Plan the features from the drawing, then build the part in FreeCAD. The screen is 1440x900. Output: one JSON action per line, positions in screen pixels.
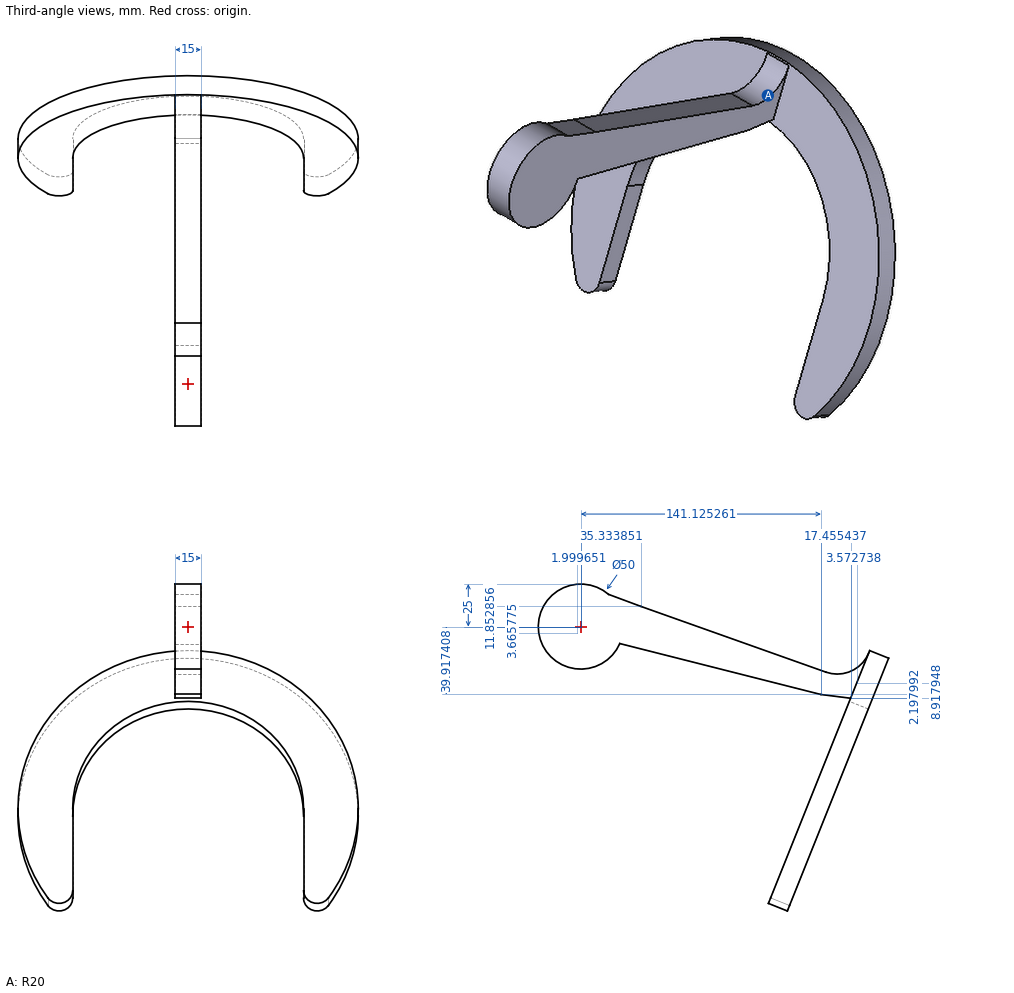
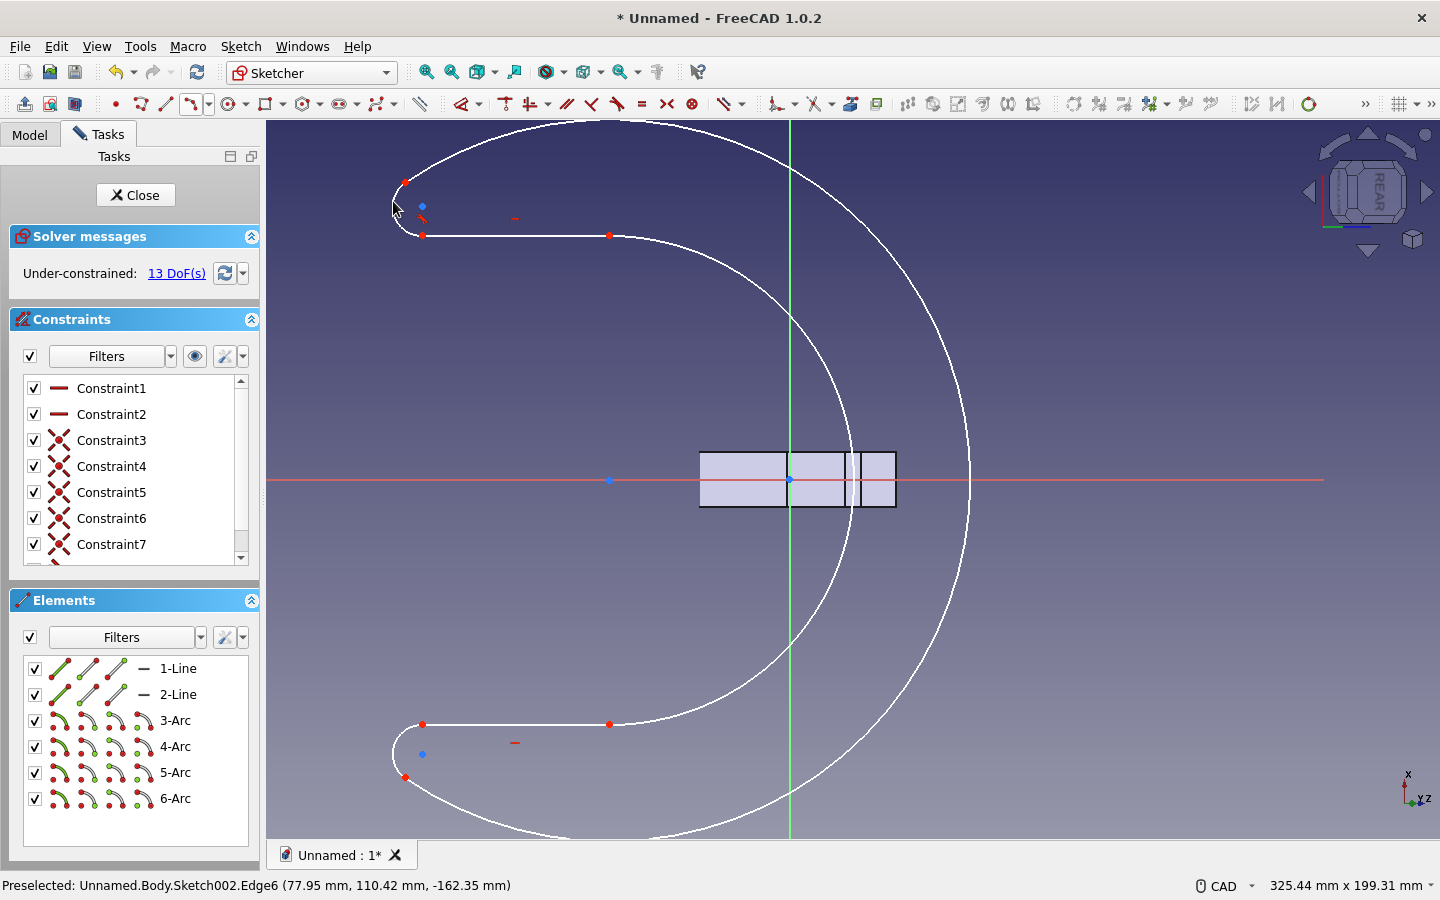
{"action": "left_click", "coordinate": [553, 725]}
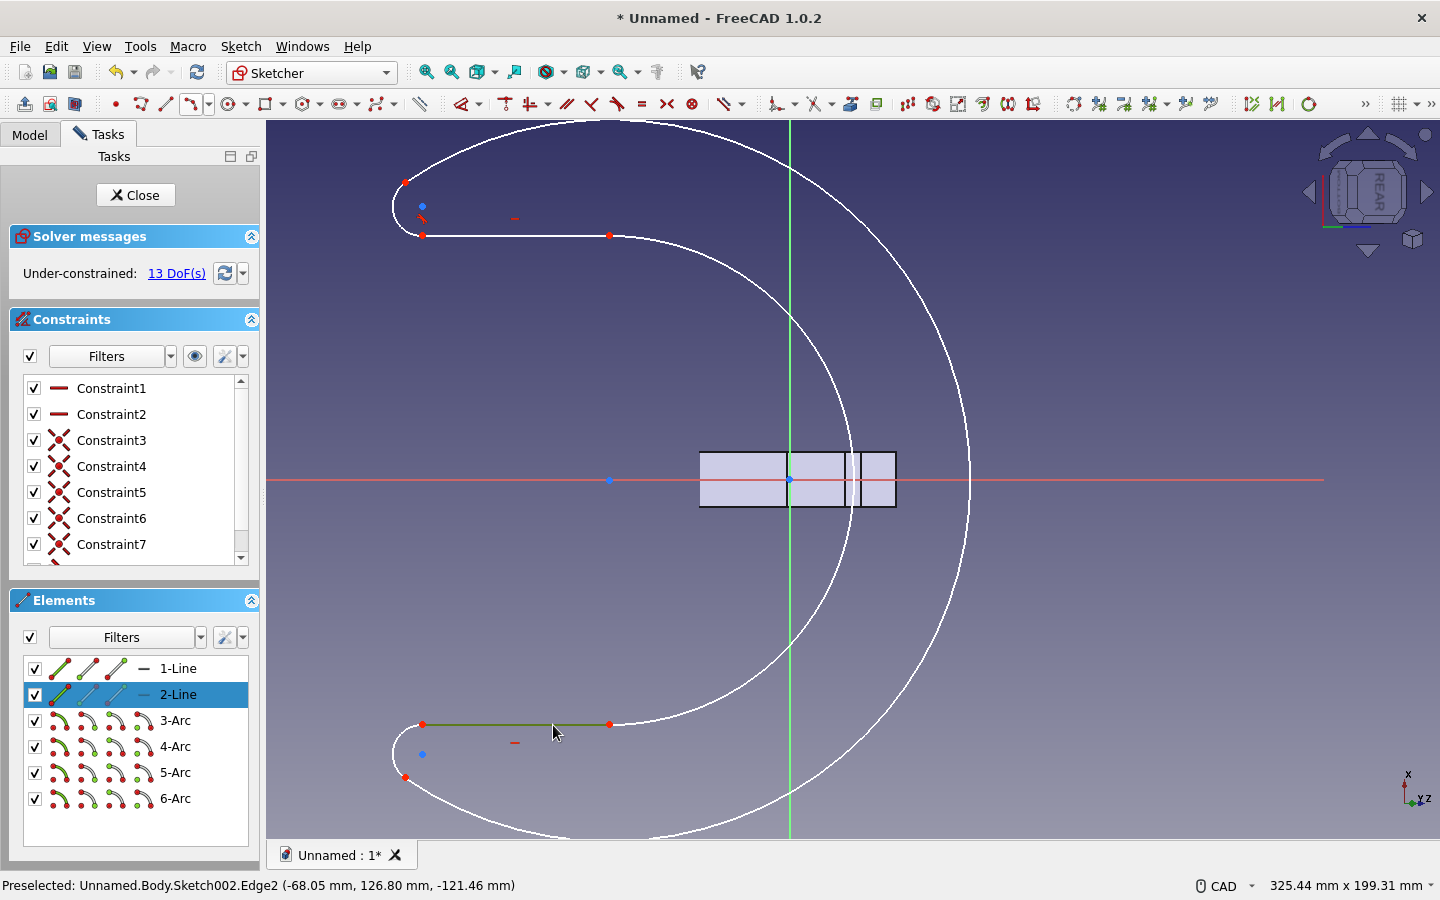
{"action": "left_click", "coordinate": [402, 733]}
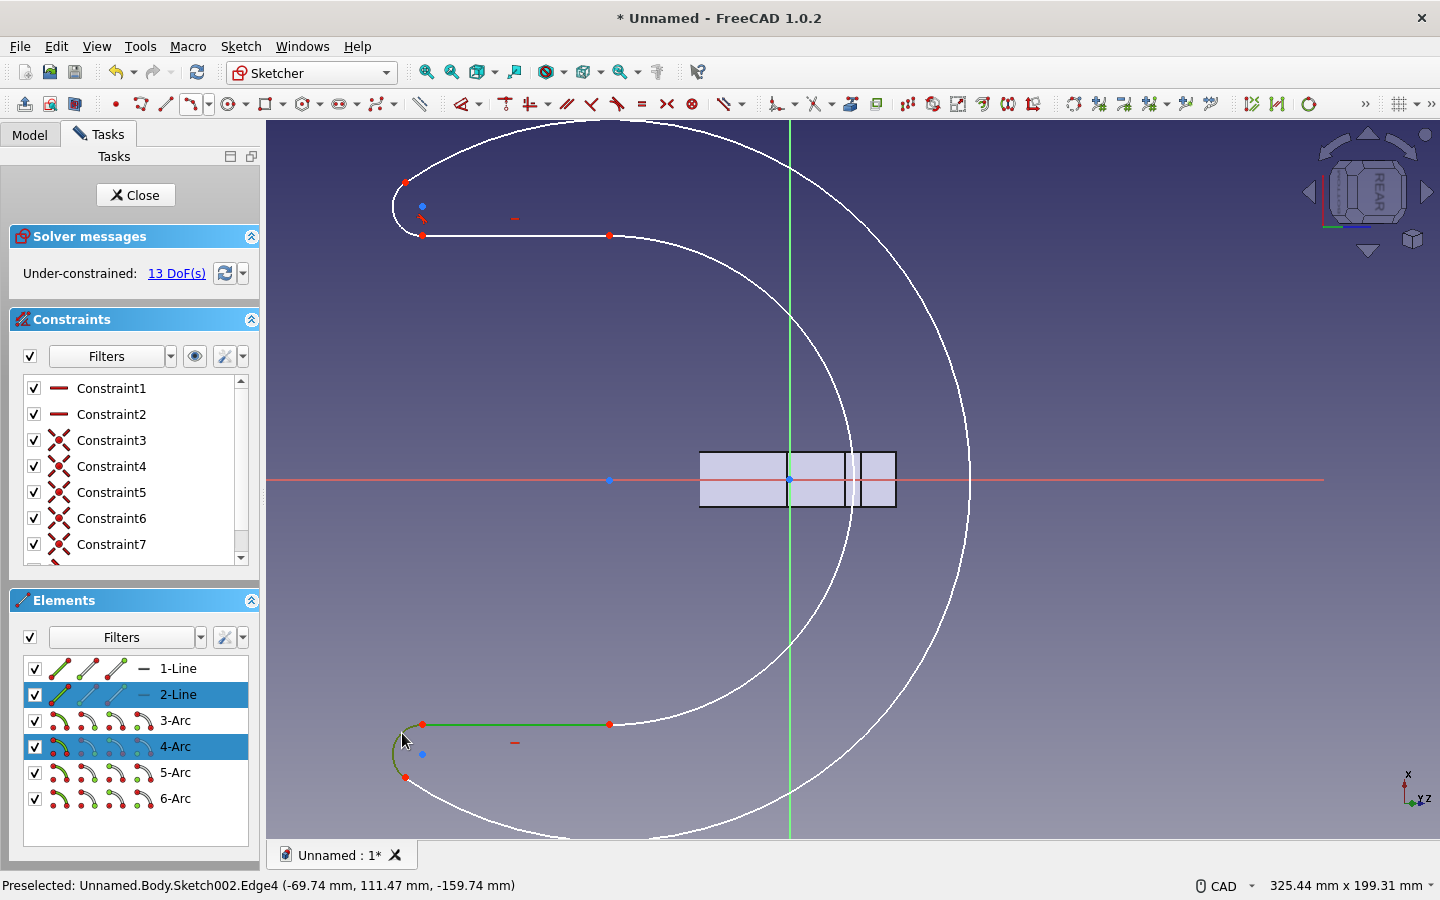
{"action": "left_click", "coordinate": [617, 104]}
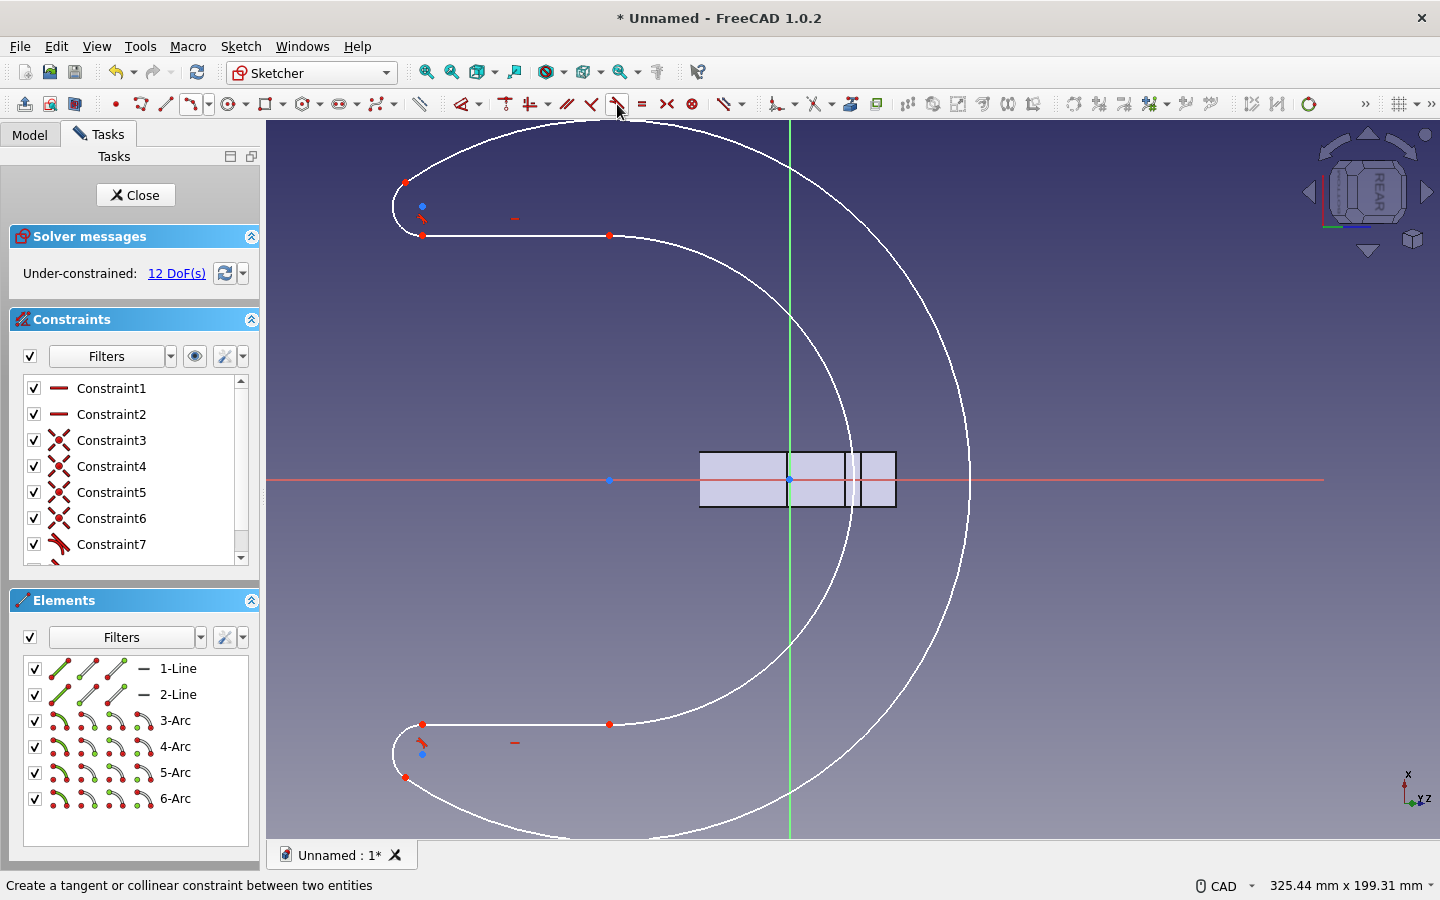
{"action": "left_click", "coordinate": [402, 733]}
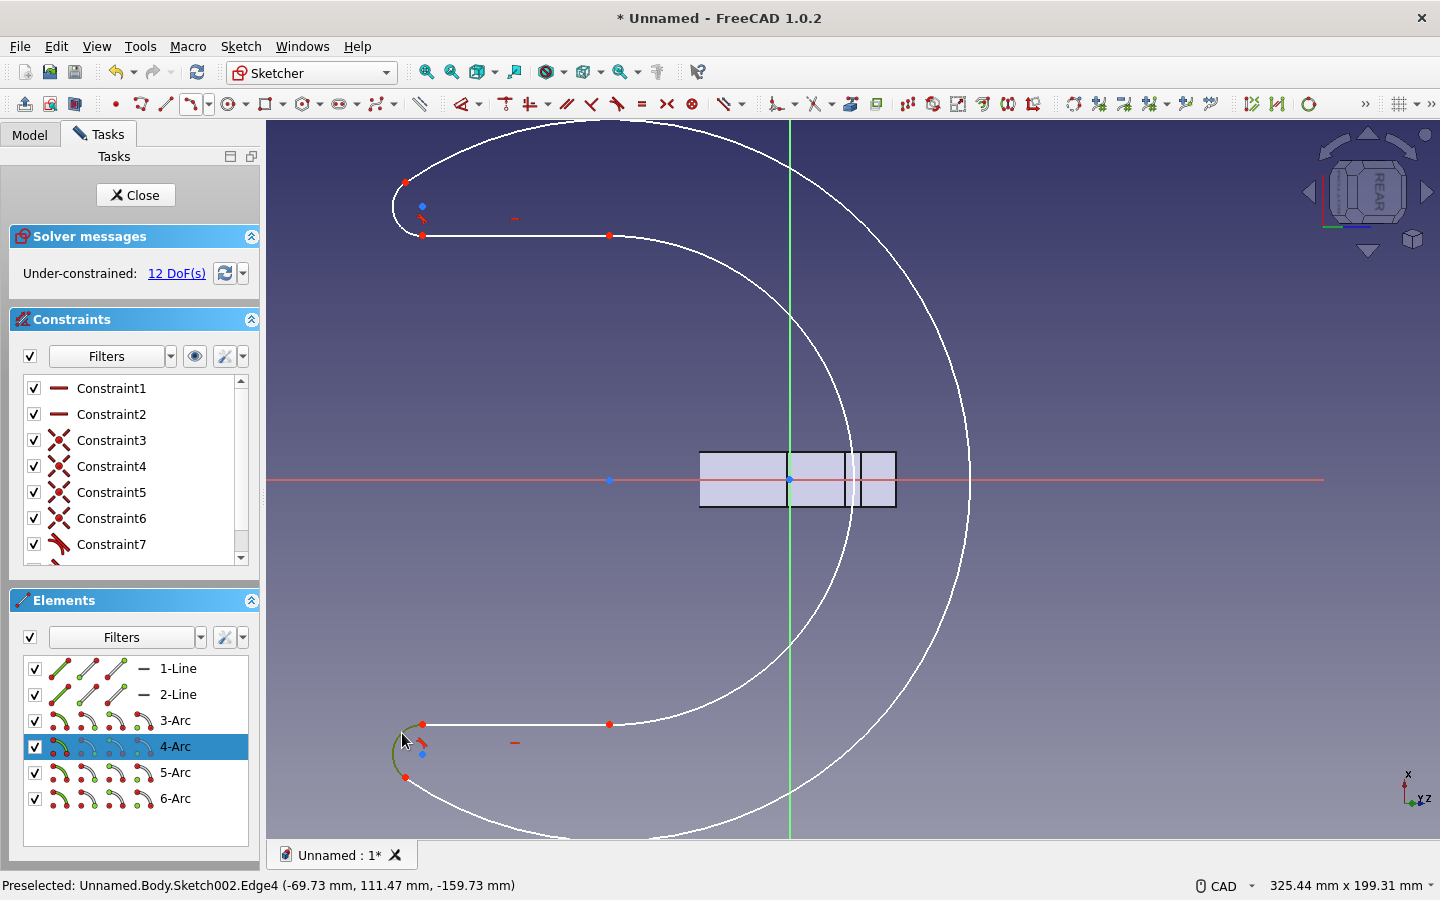
{"action": "left_click", "coordinate": [842, 756]}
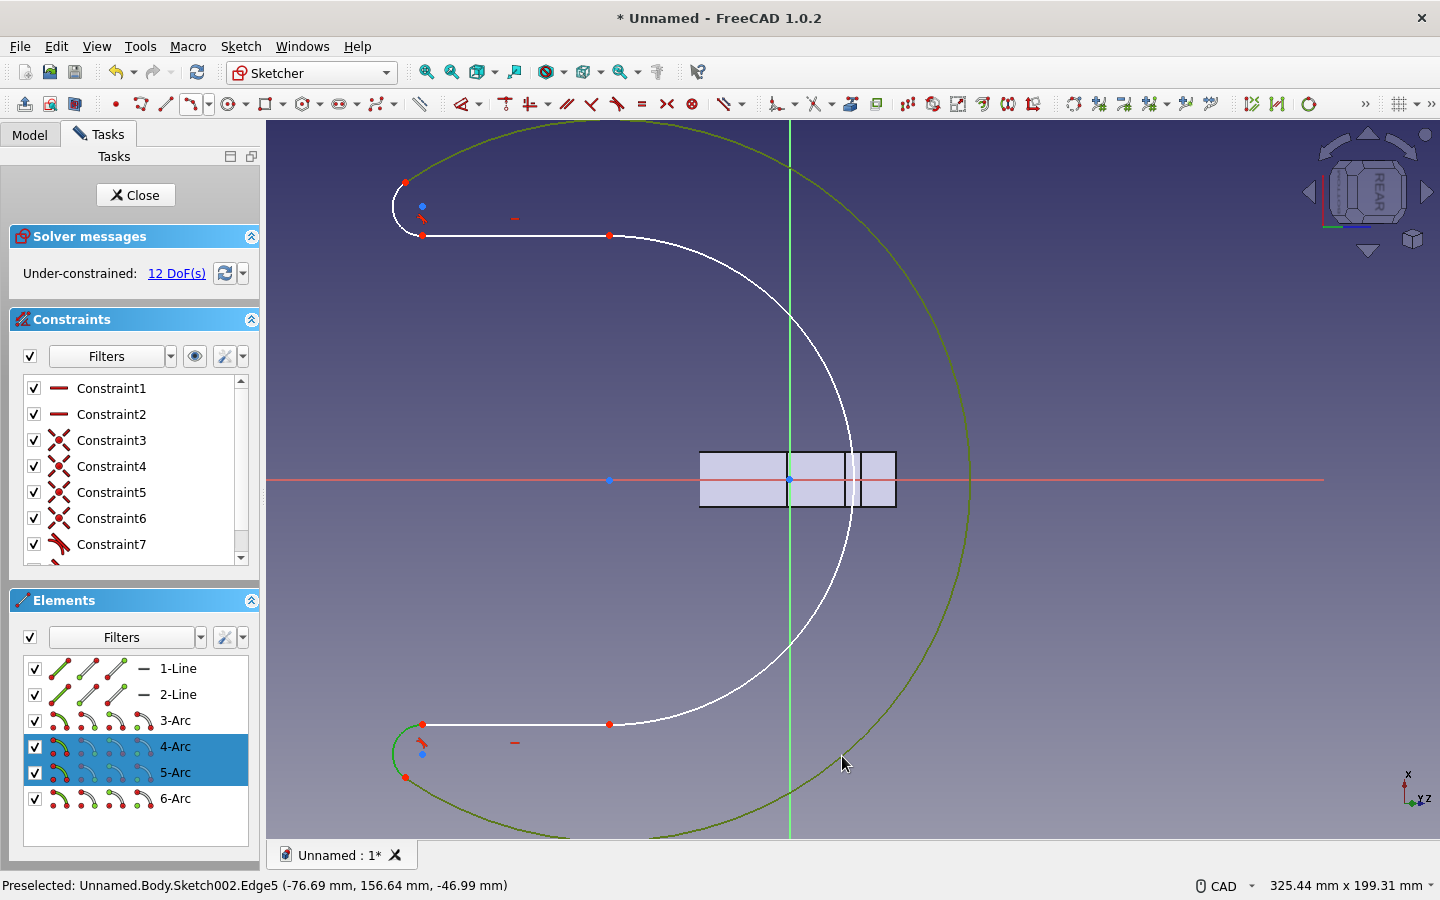
{"action": "left_click", "coordinate": [617, 104]}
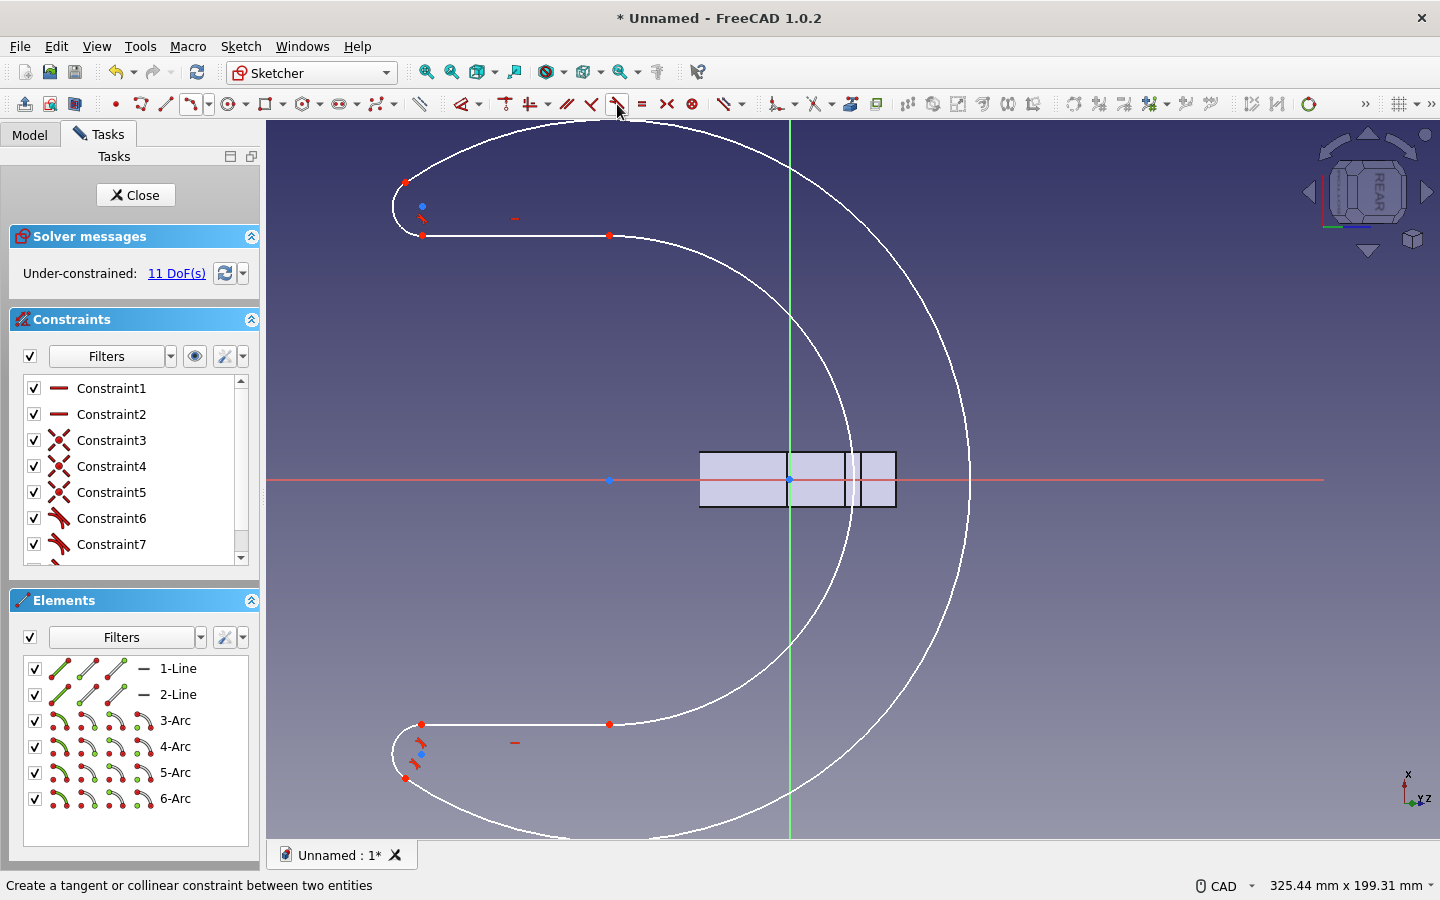
{"action": "left_click", "coordinate": [842, 756]}